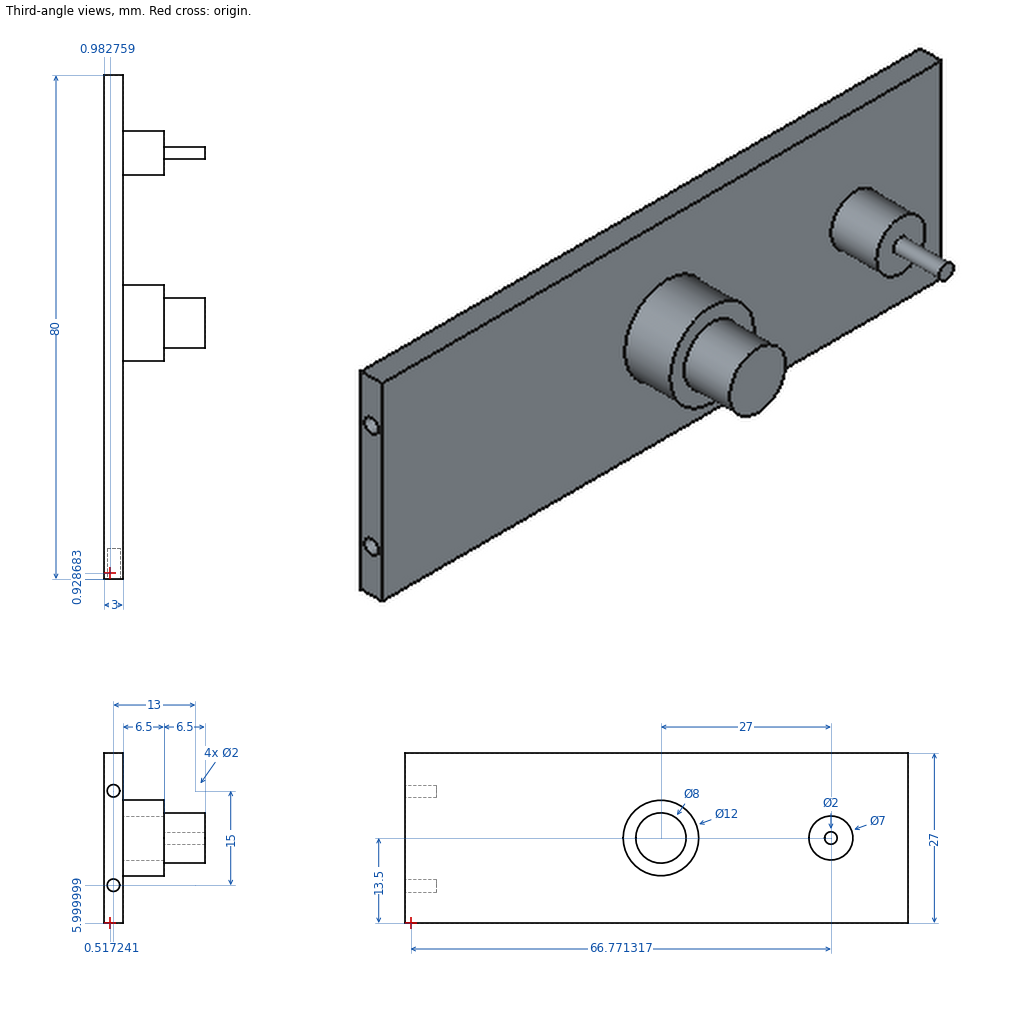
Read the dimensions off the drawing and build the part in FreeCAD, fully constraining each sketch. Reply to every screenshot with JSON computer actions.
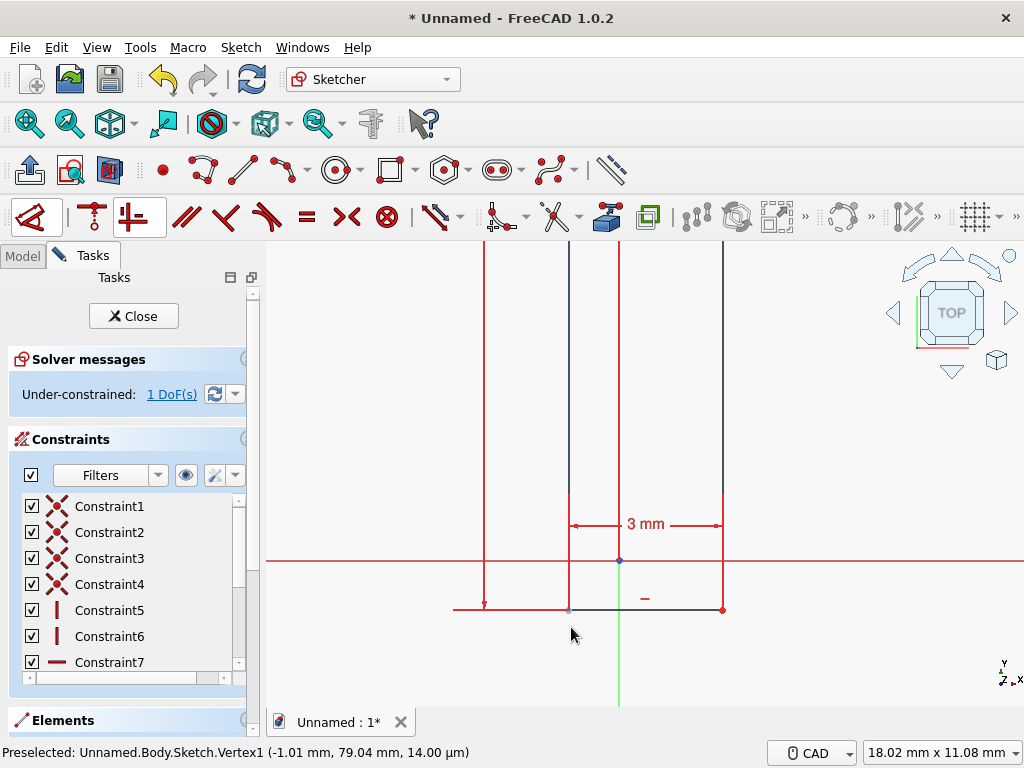
{"action": "left_click", "coordinate": [569, 610]}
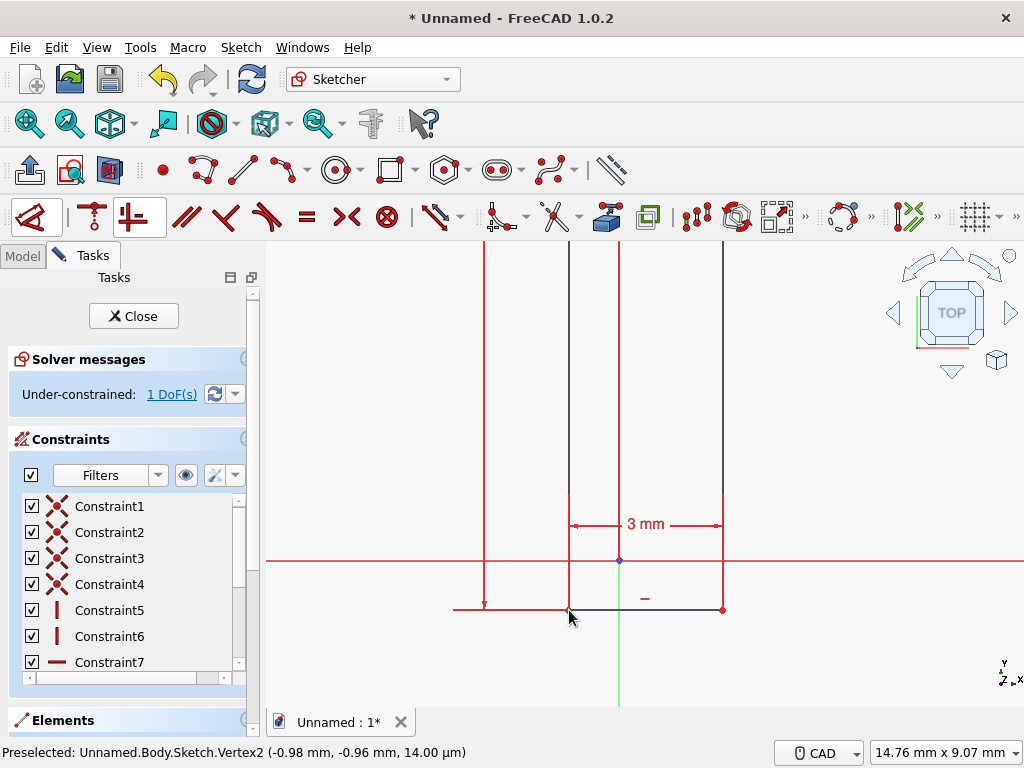
{"action": "key", "text": "i"}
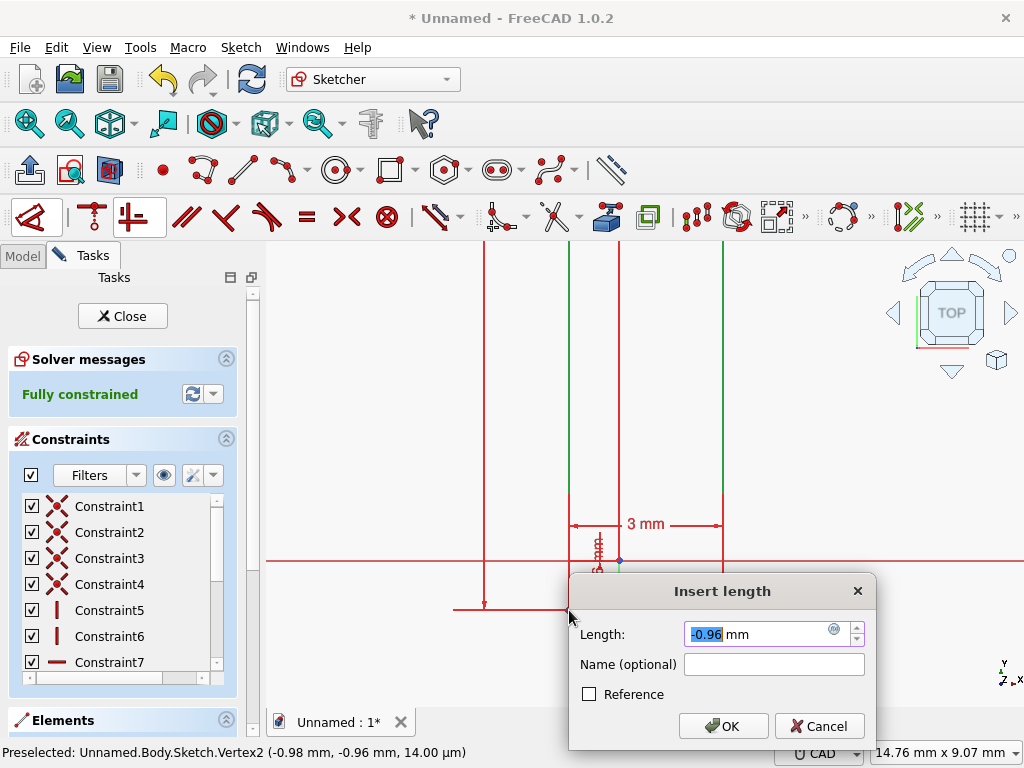
{"action": "type", "text": "-0.928683"}
{"action": "key", "text": "Return"}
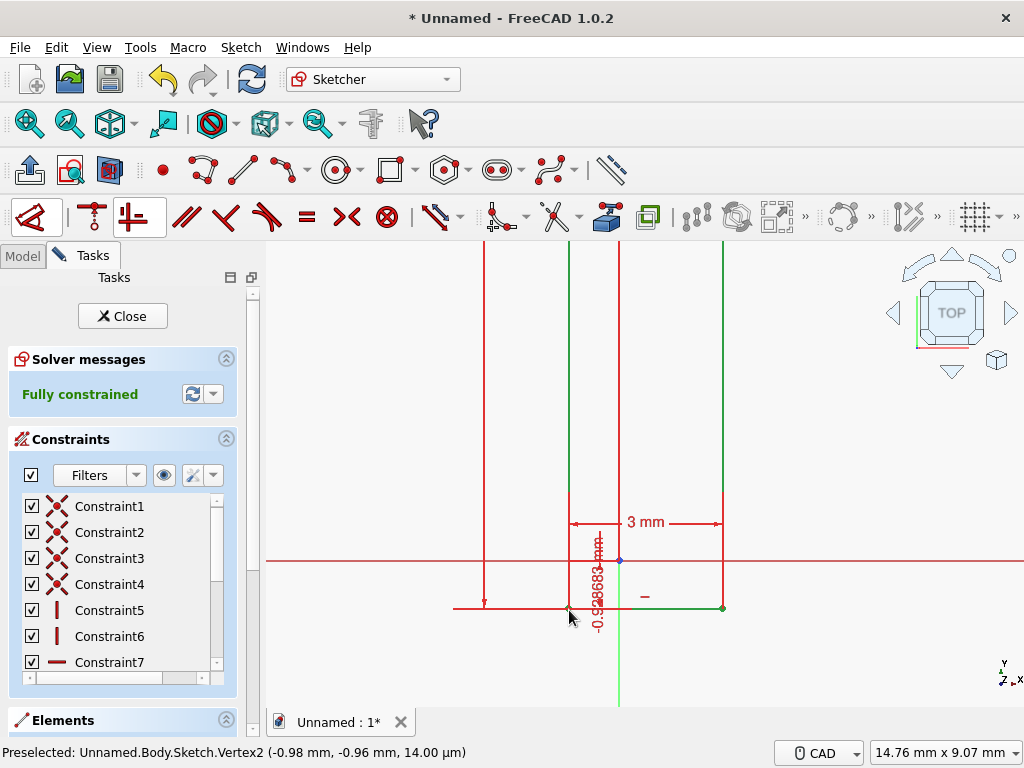
{"action": "left_click", "coordinate": [123, 316]}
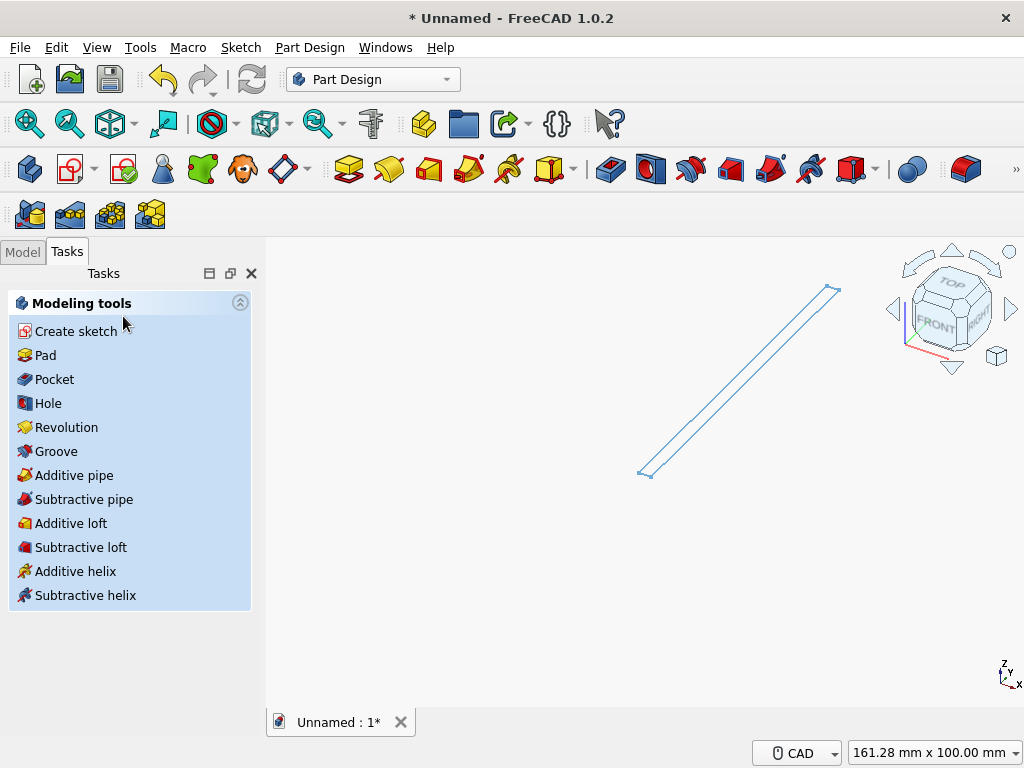
{"action": "left_click", "coordinate": [350, 170]}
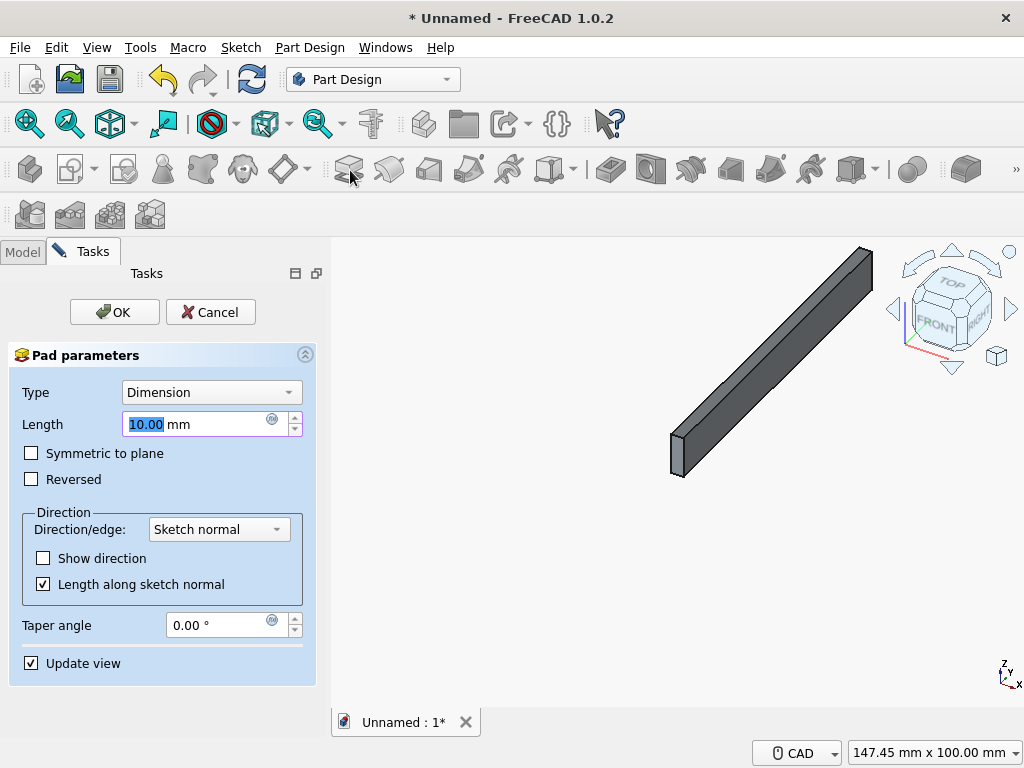
{"action": "type", "text": "27"}
{"action": "key", "text": "Tab"}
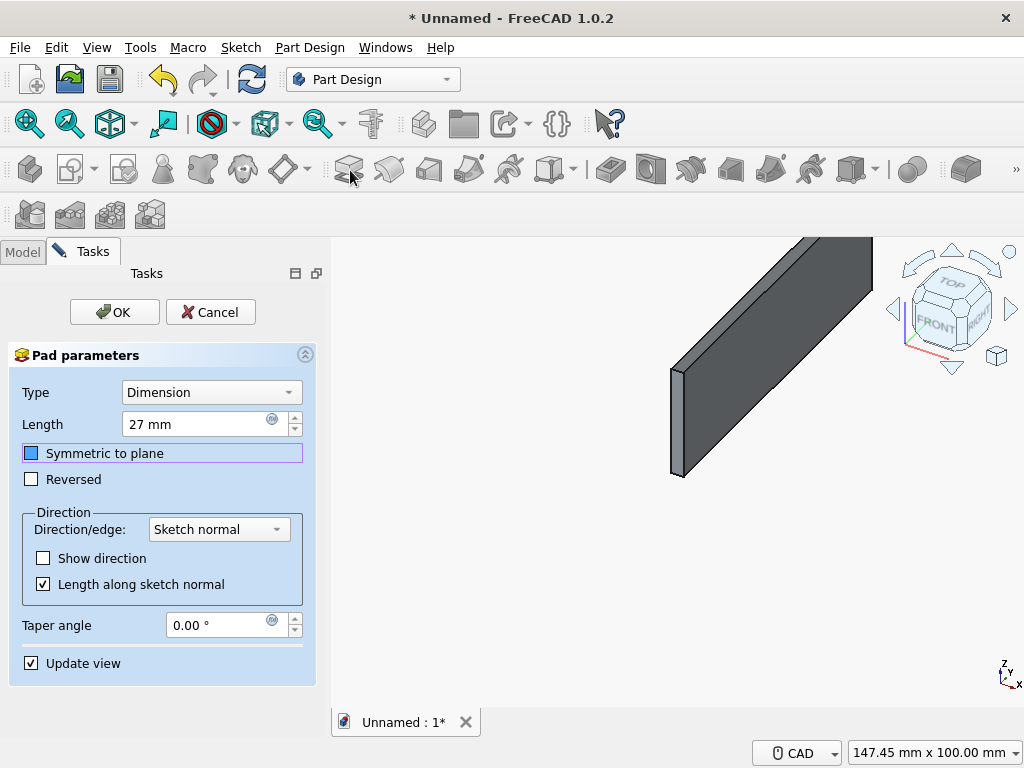
{"action": "left_click", "coordinate": [115, 312]}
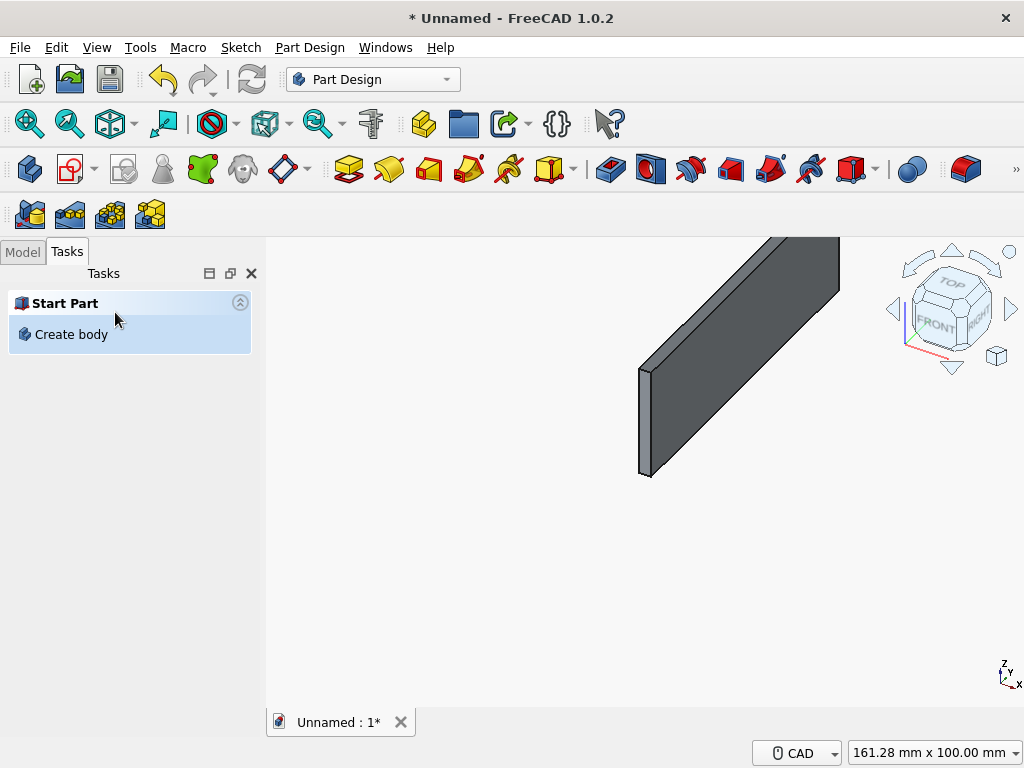
{"action": "left_click", "coordinate": [30, 124]}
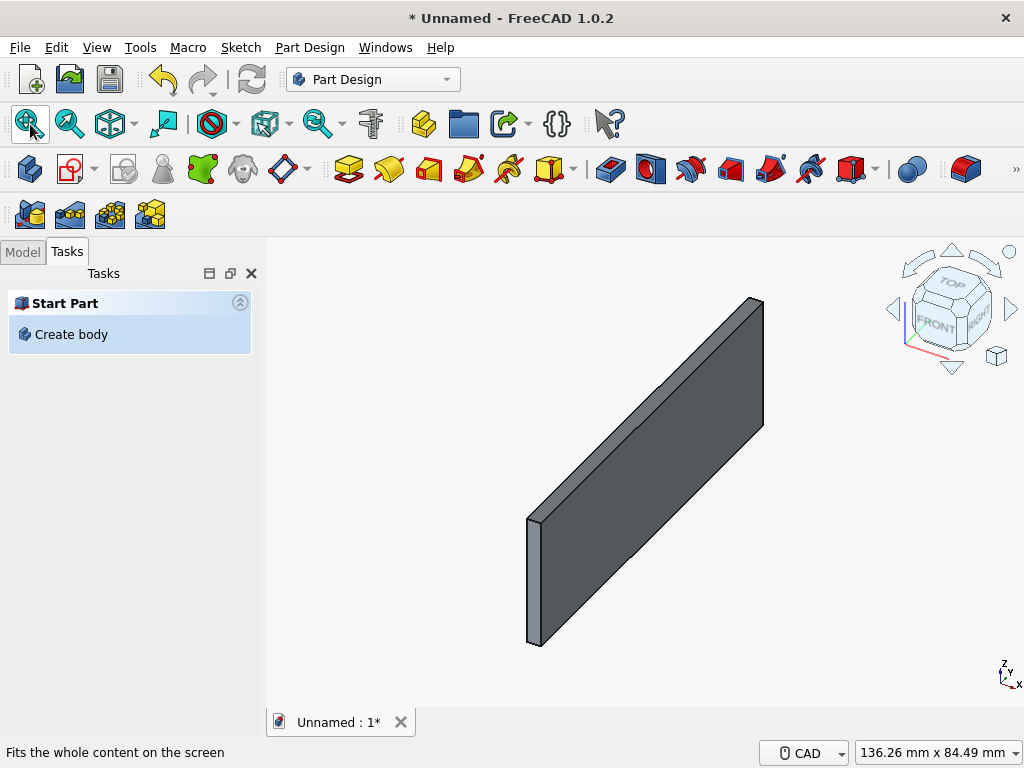
{"action": "left_click", "coordinate": [716, 410]}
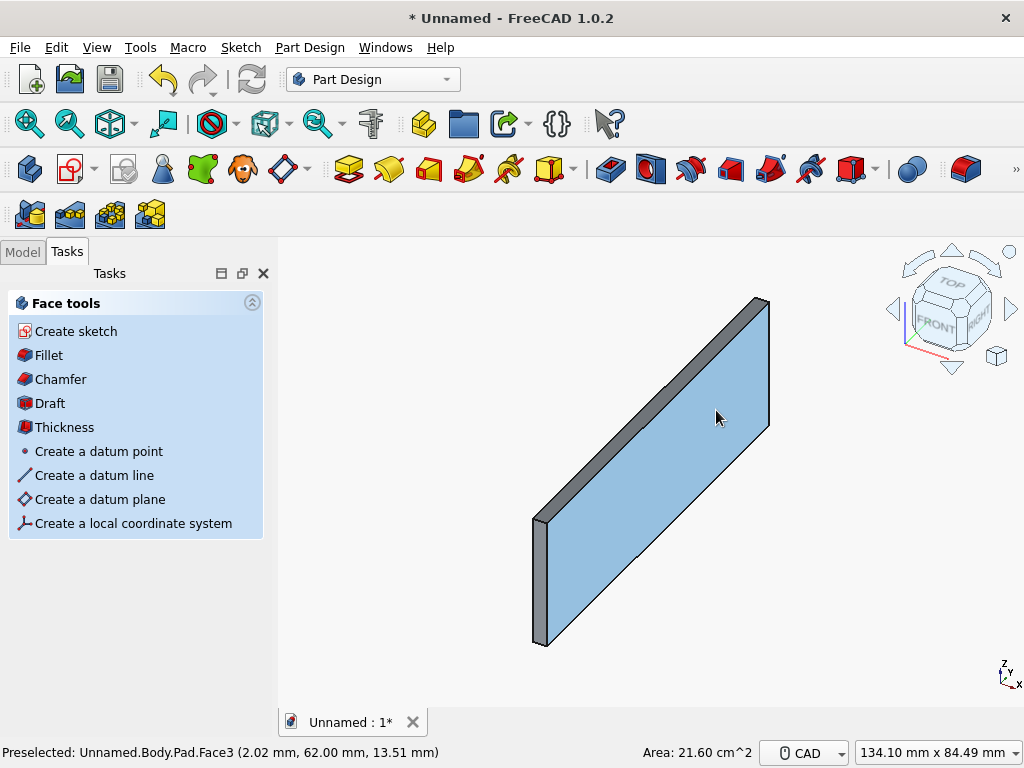
{"action": "left_click", "coordinate": [70, 170]}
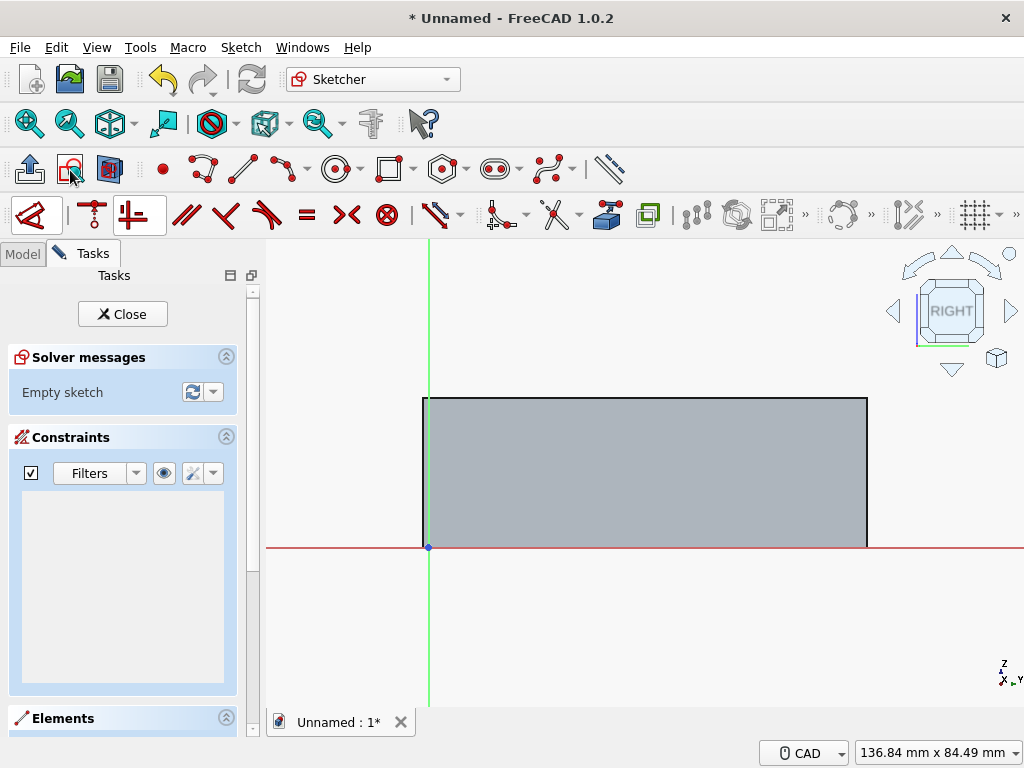
{"action": "left_click", "coordinate": [336, 170]}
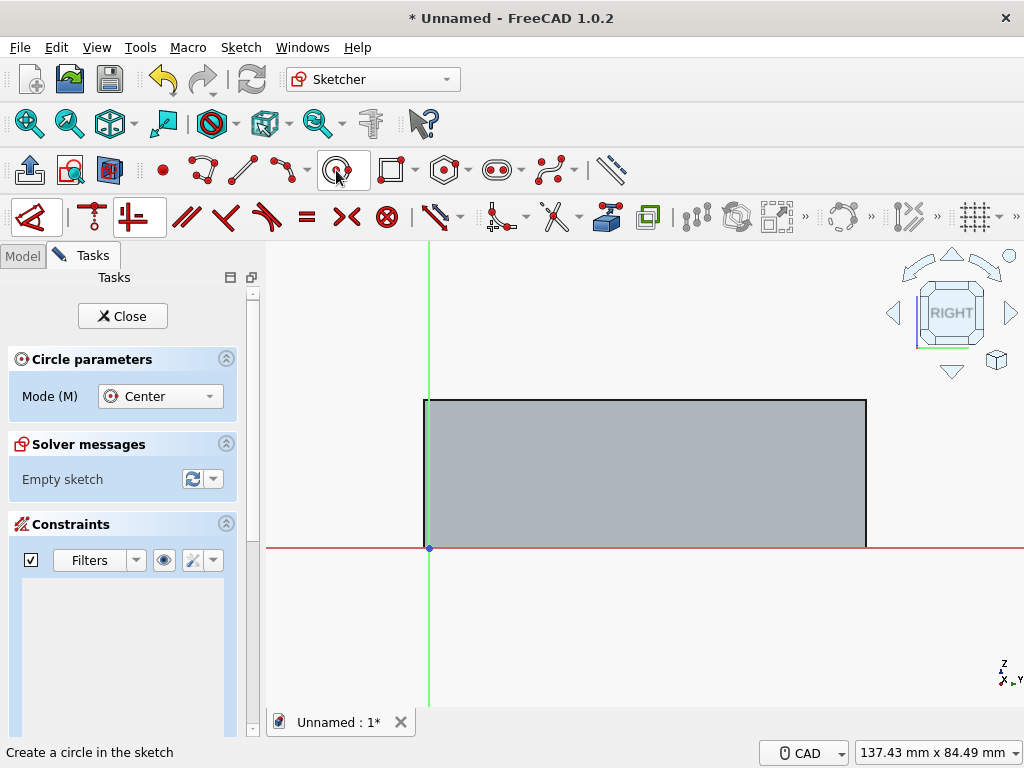
{"action": "left_click", "coordinate": [798, 474]}
{"action": "mouse_move", "coordinate": [811, 460]}